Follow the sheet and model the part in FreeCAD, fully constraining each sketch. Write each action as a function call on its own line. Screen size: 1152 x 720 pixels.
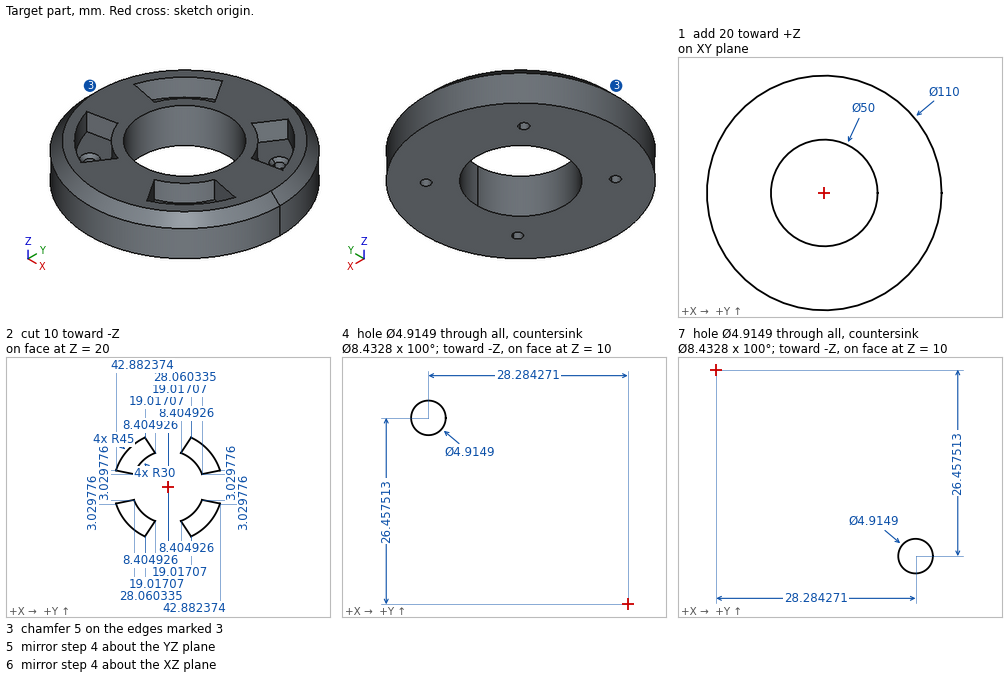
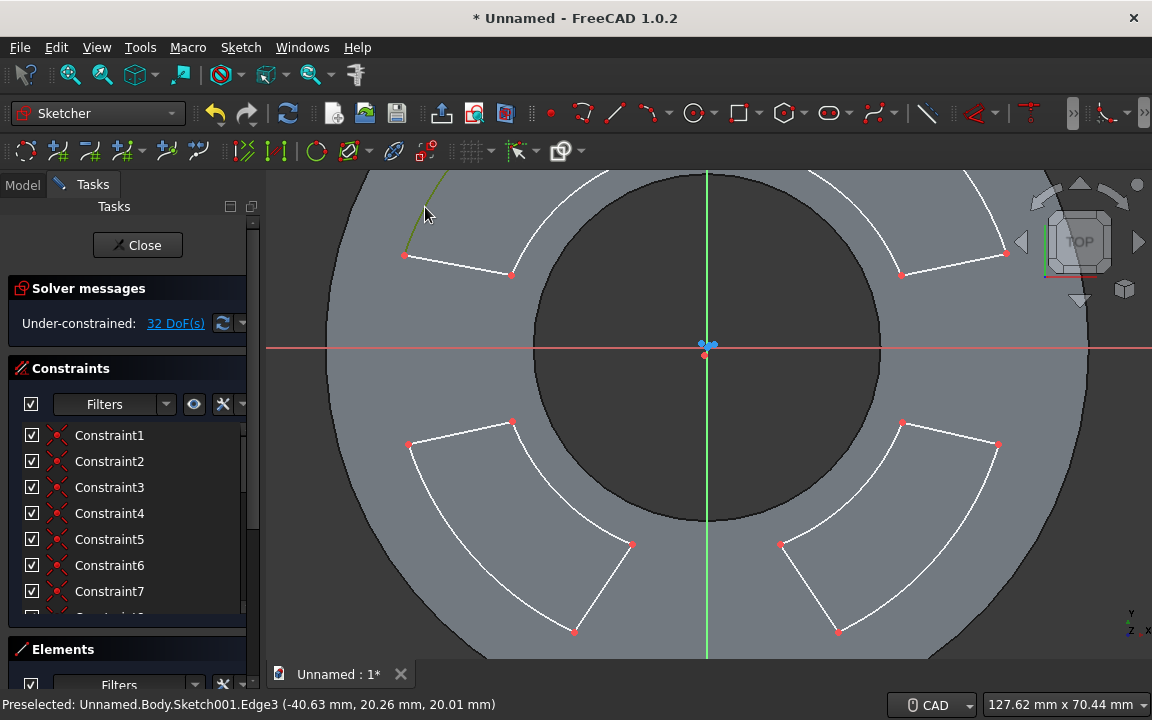
click(827, 519)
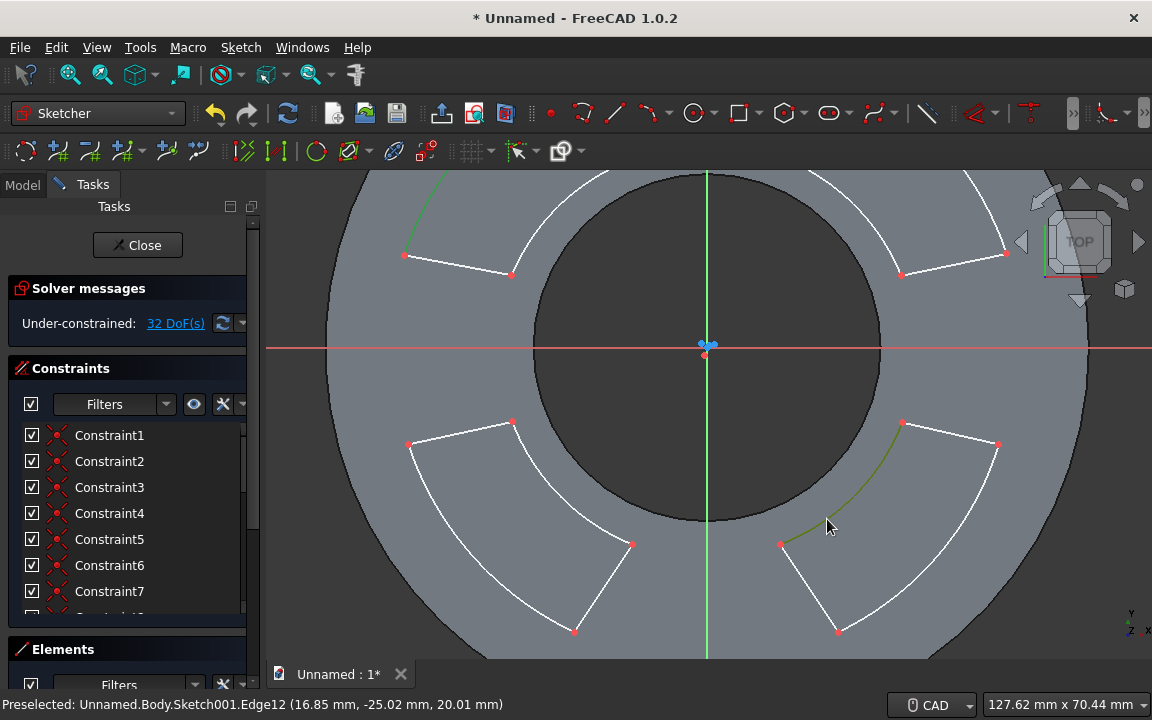
click(1030, 114)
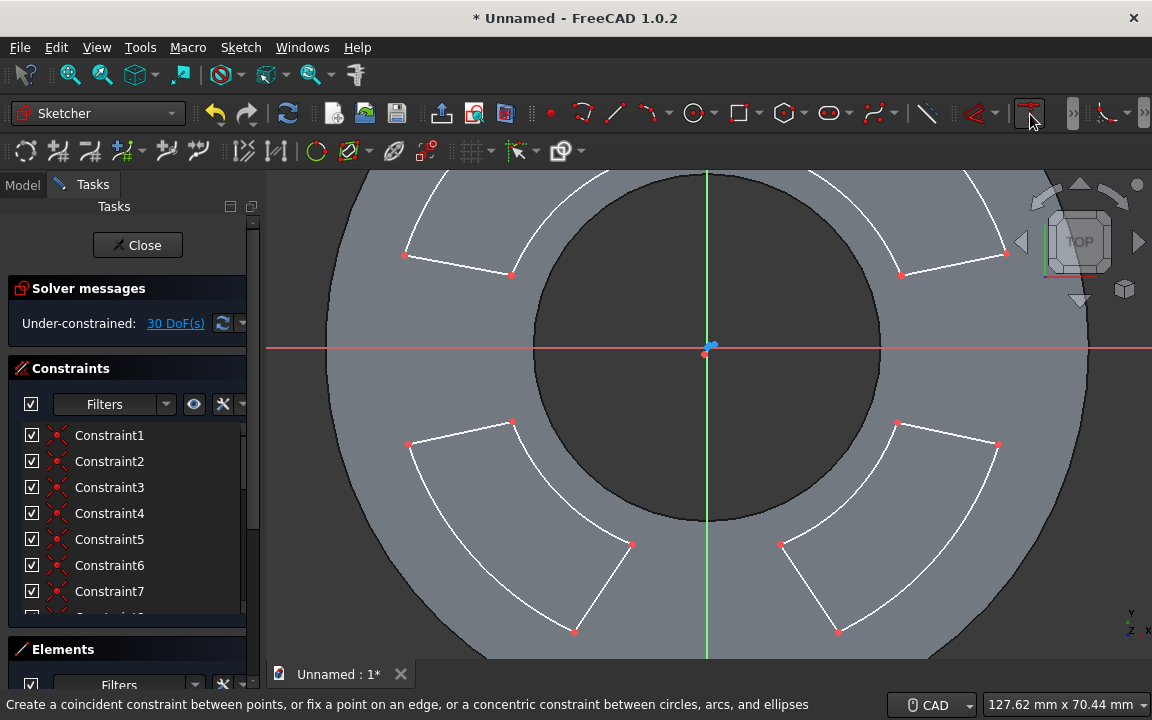
click(425, 207)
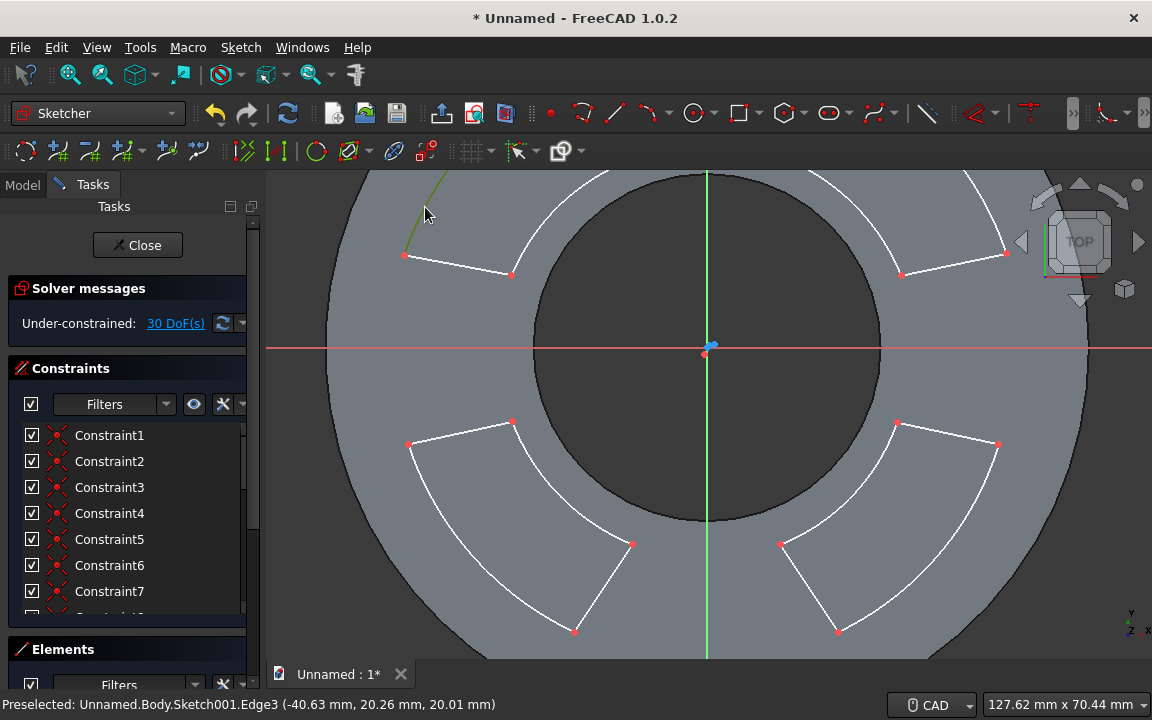
click(441, 514)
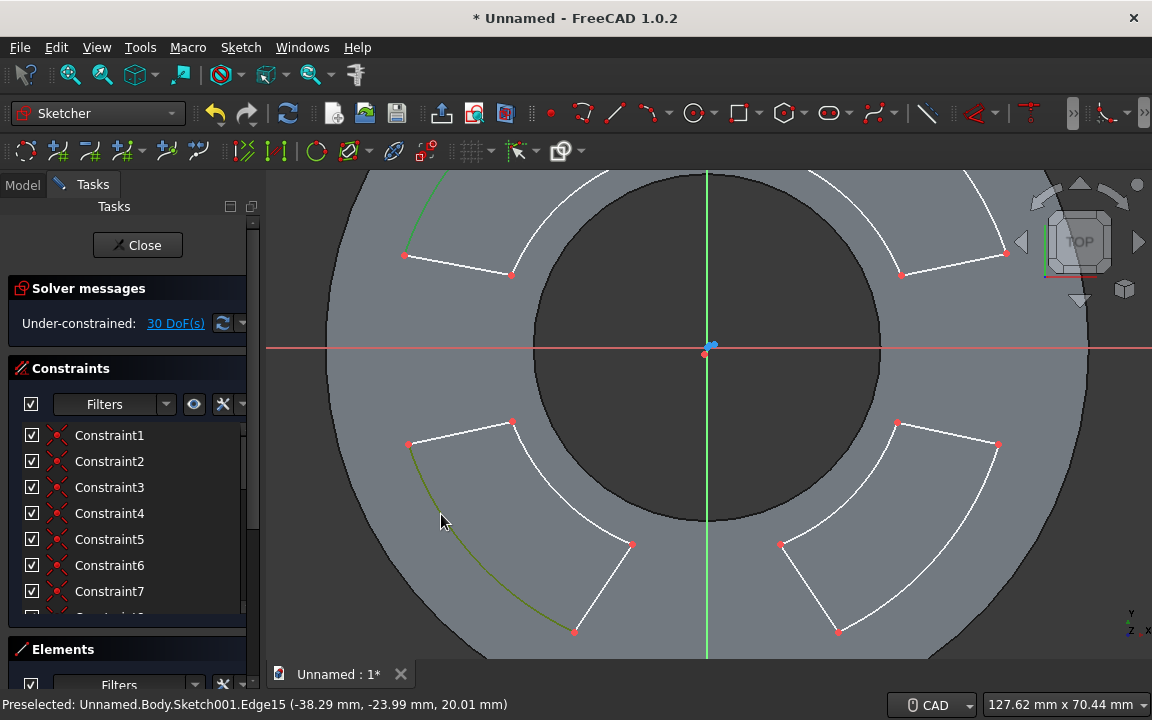
click(1030, 114)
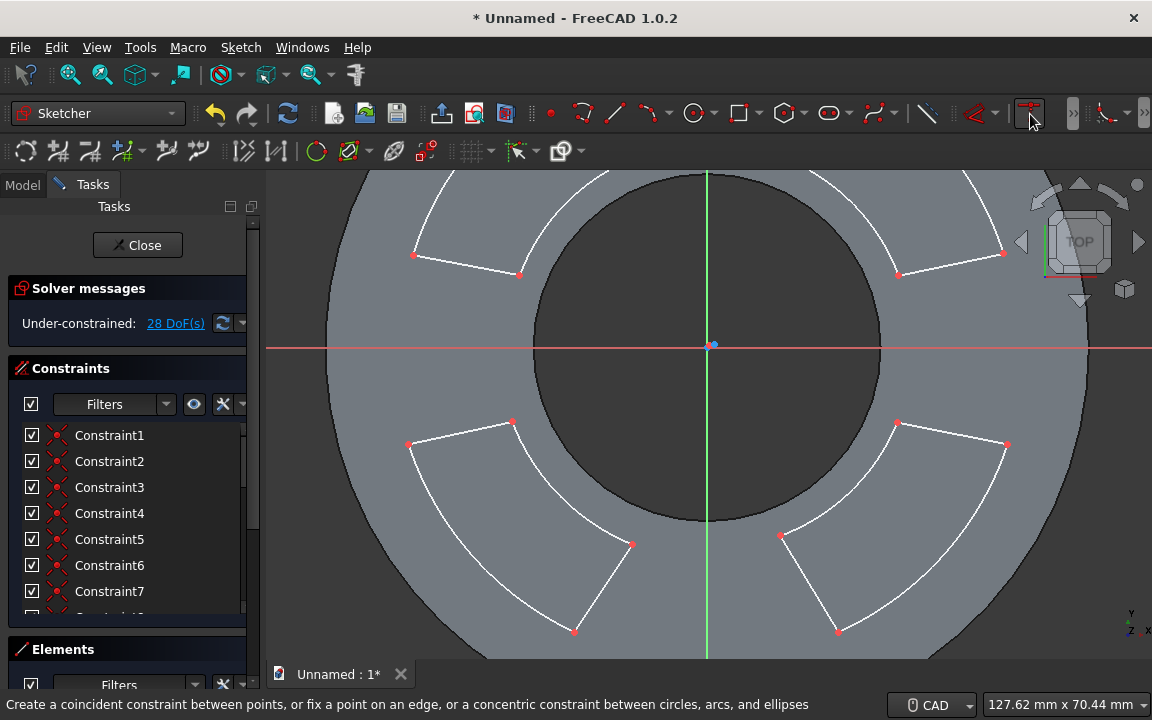
click(432, 208)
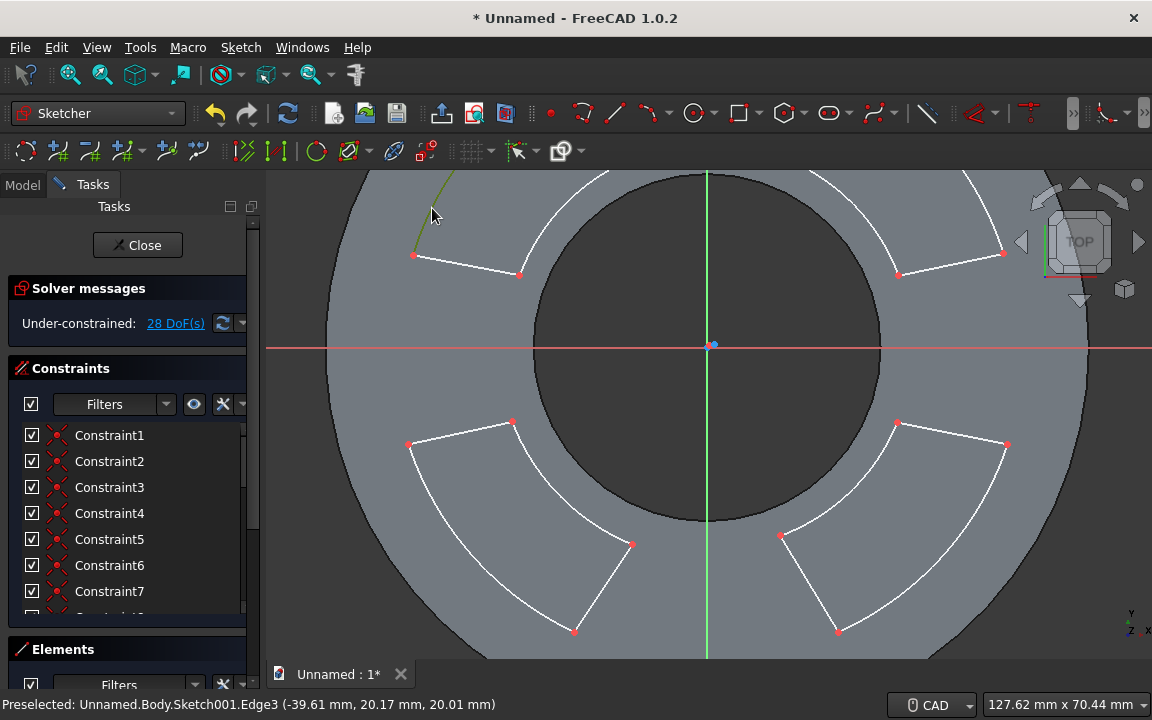
click(537, 469)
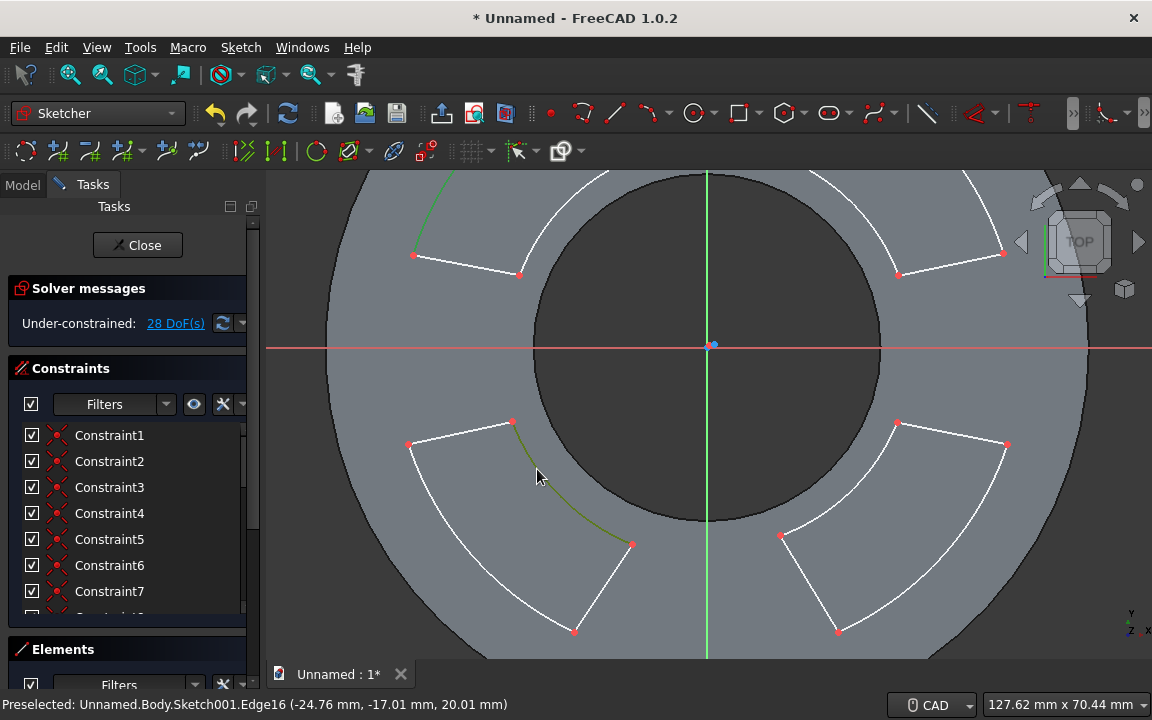
click(1030, 114)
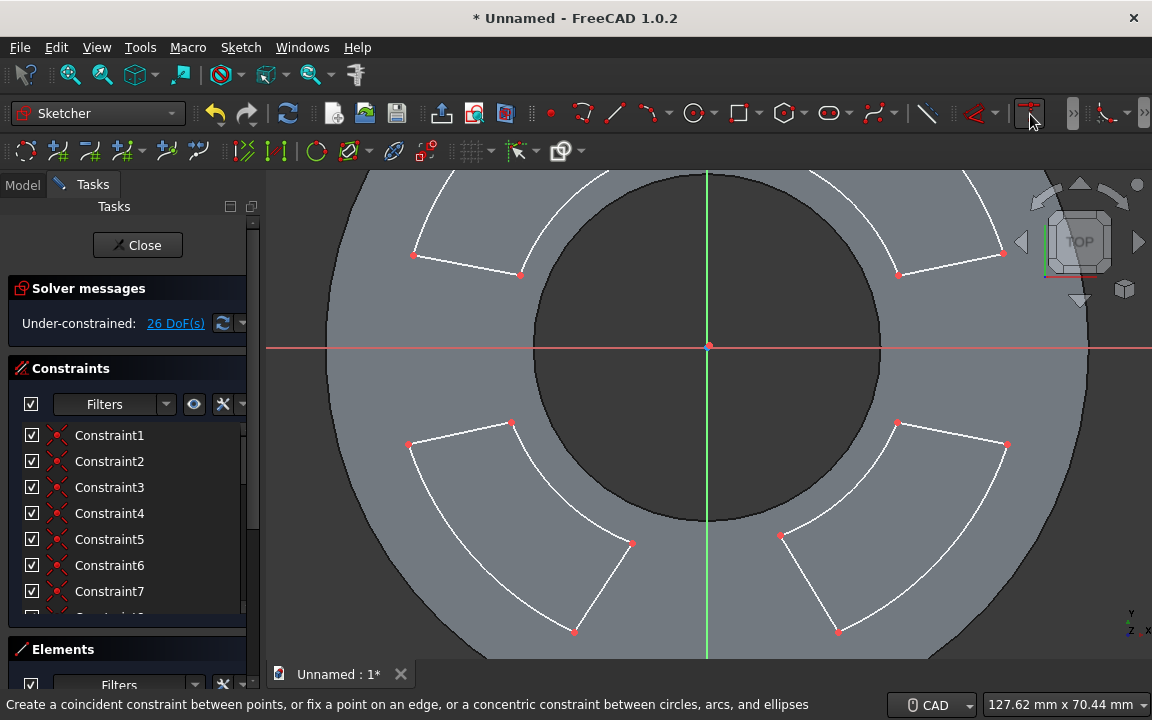
drag(697, 336, 720, 358)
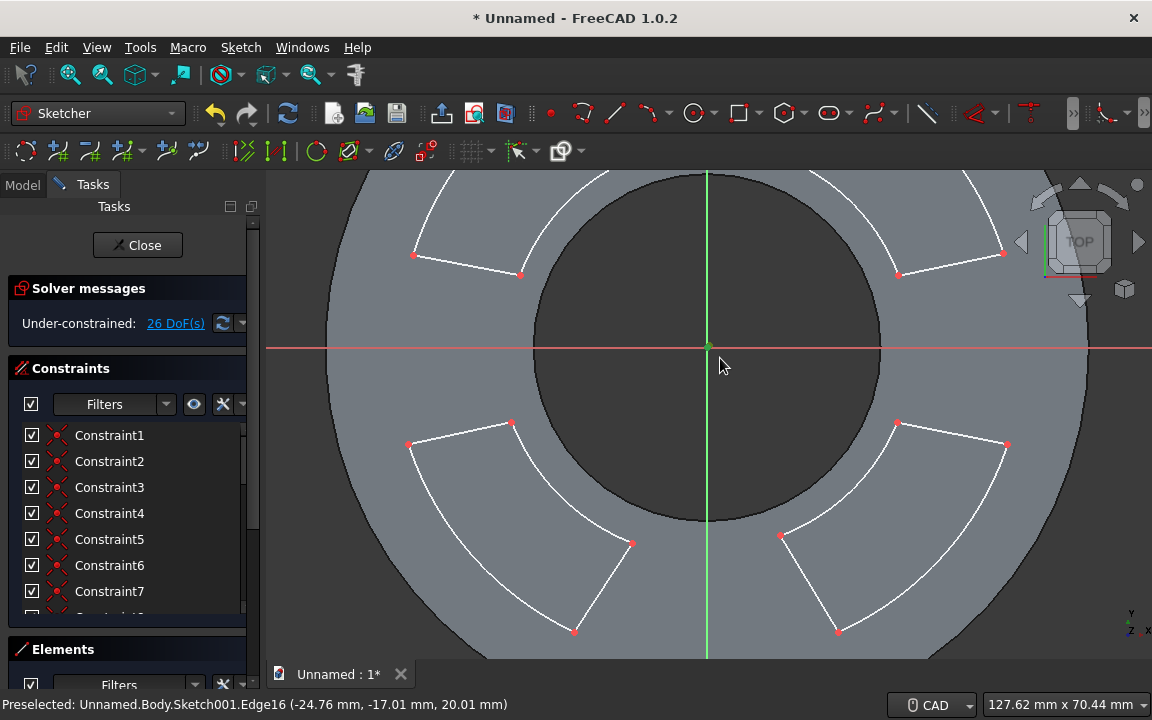
click(1030, 114)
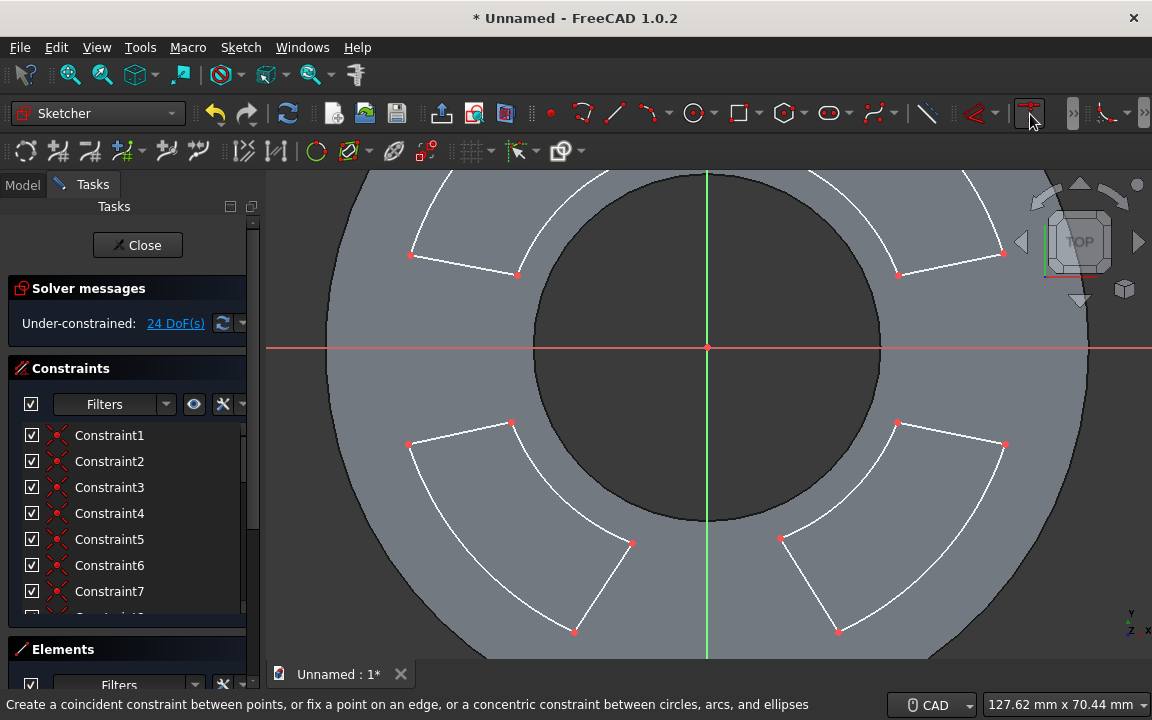
click(430, 207)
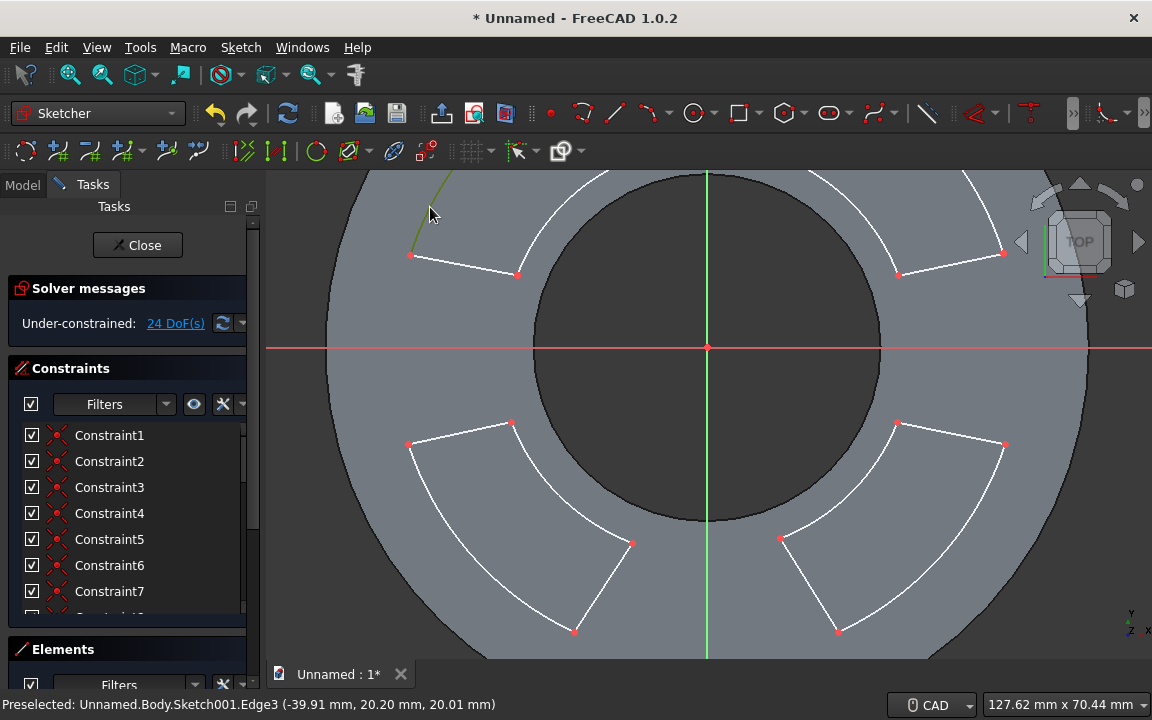
click(984, 206)